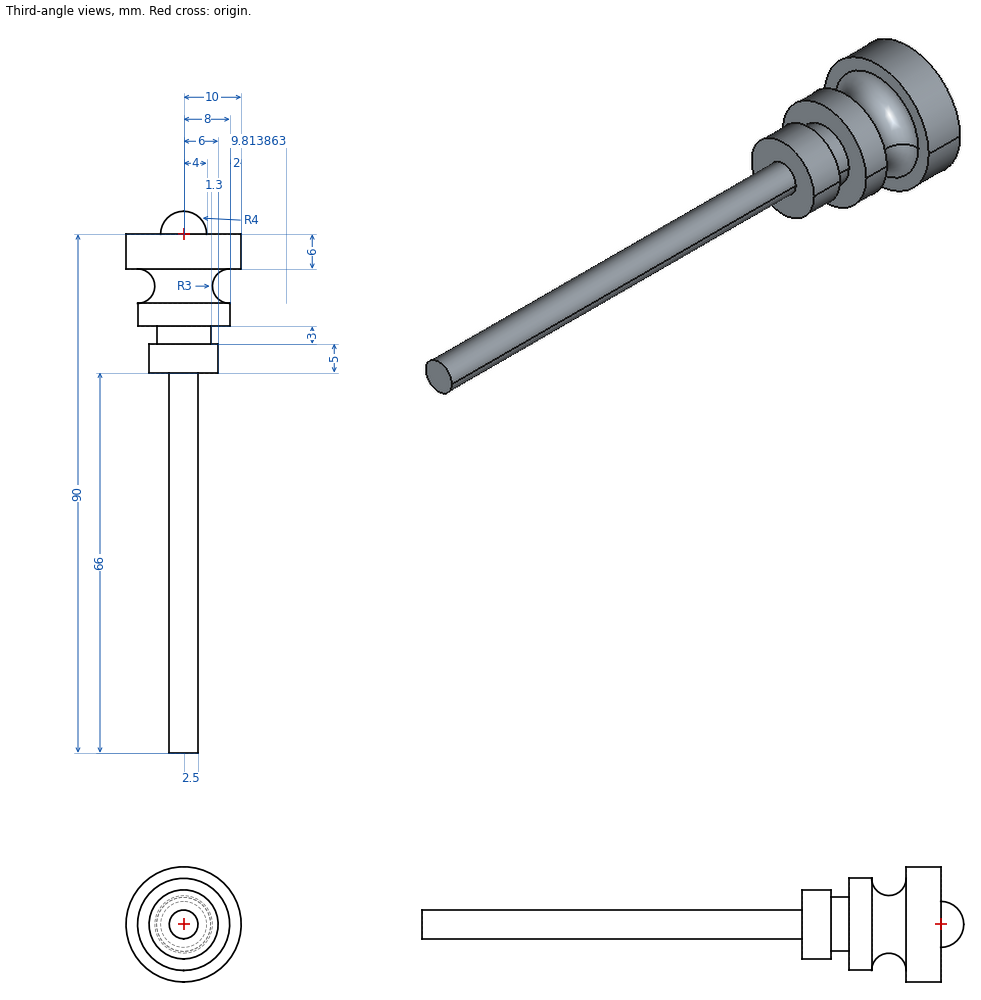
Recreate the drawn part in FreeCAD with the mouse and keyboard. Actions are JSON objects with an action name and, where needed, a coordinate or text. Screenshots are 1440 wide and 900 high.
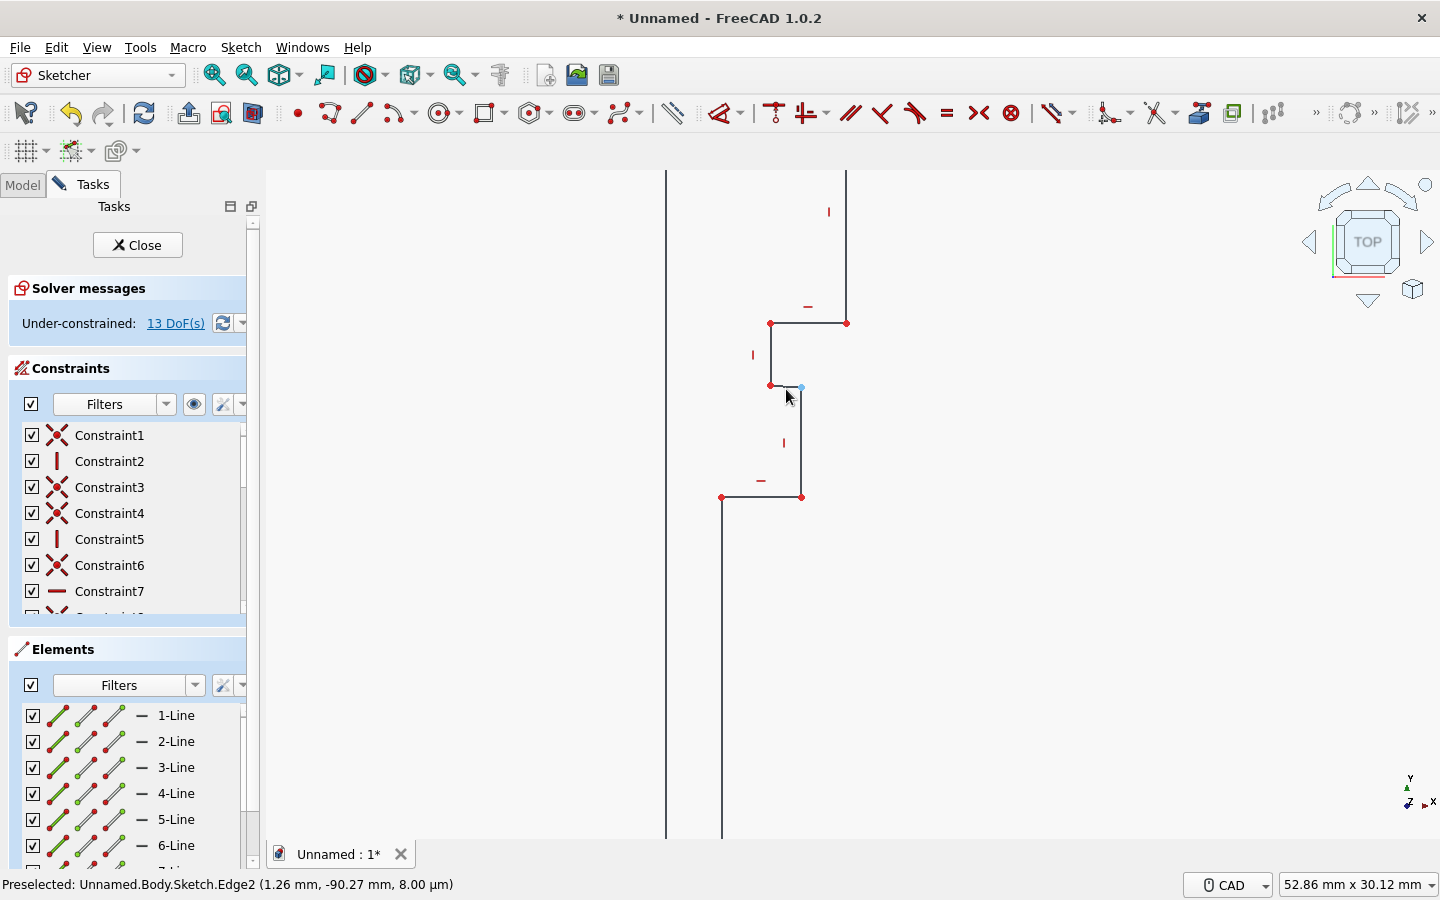
{"action": "left_click", "coordinate": [786, 387]}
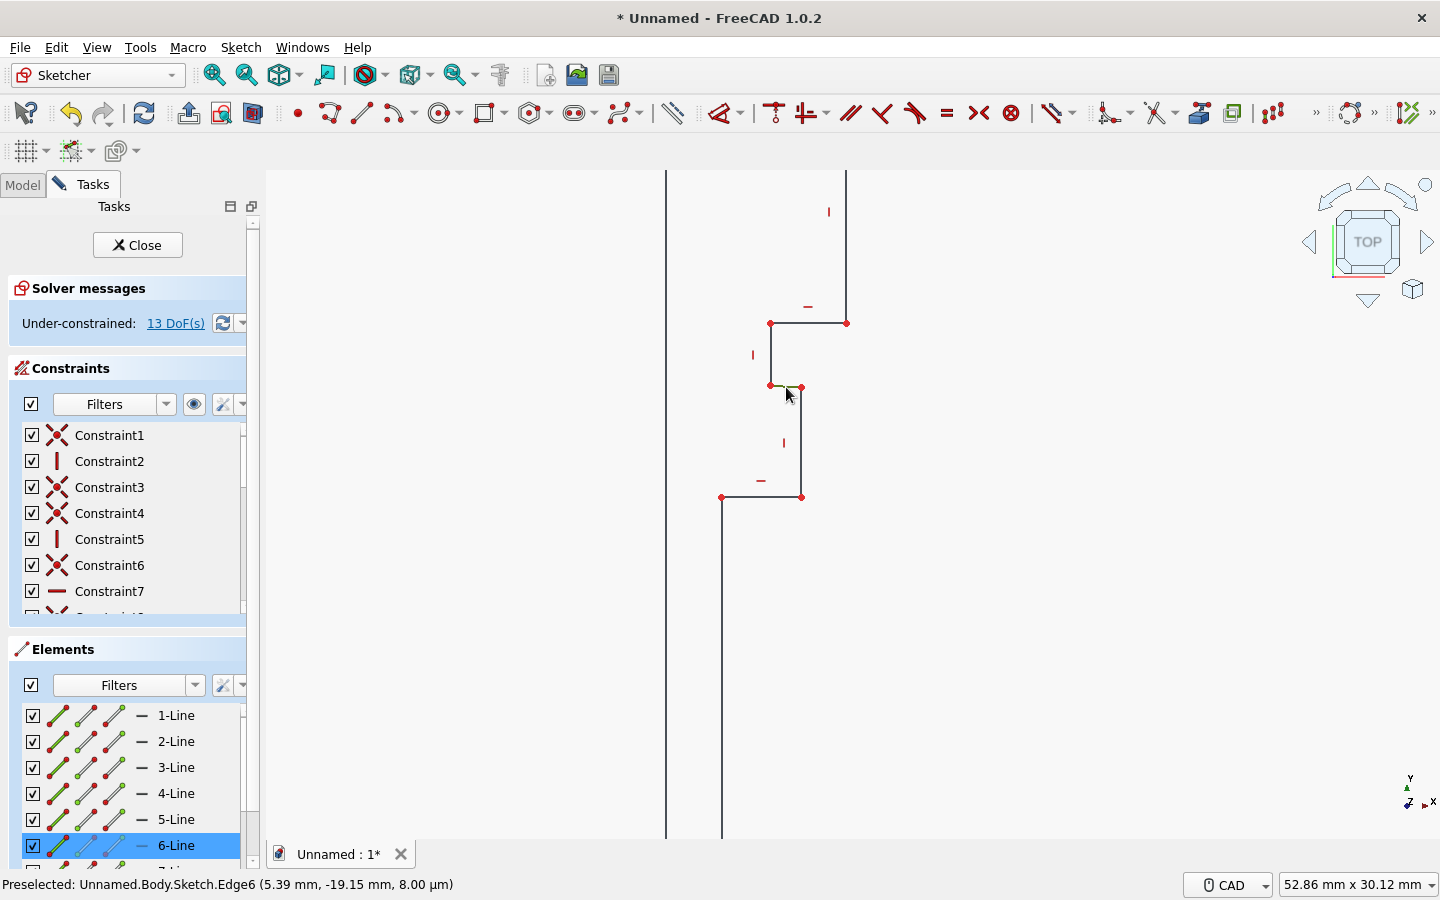
{"action": "left_click", "coordinate": [828, 114]}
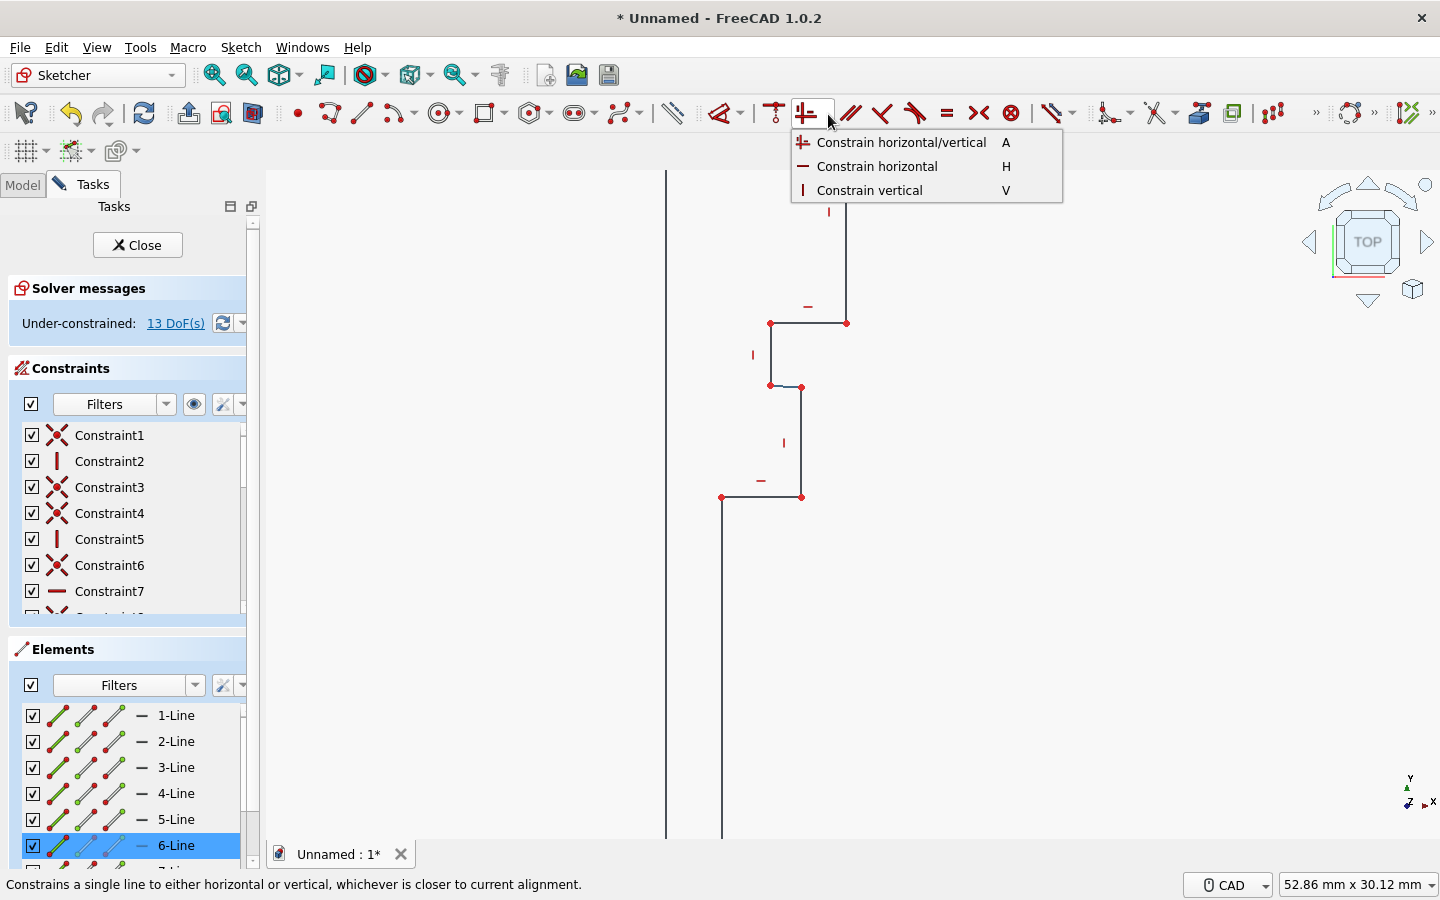
{"action": "left_click", "coordinate": [927, 166]}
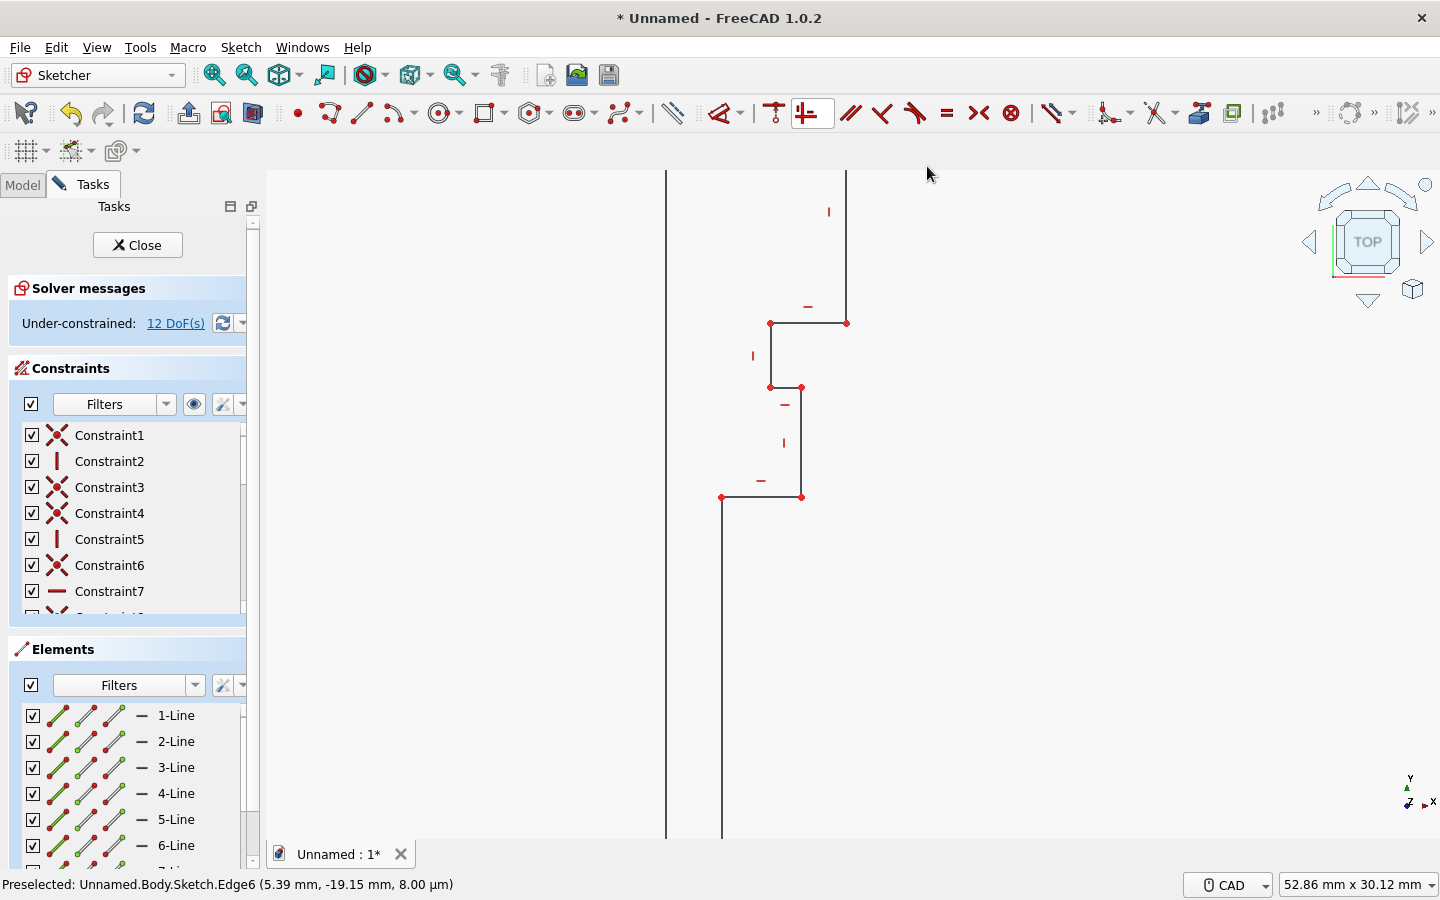
{"action": "scroll", "coordinate": [786, 389], "scroll_direction": "down", "scroll_amount": 8}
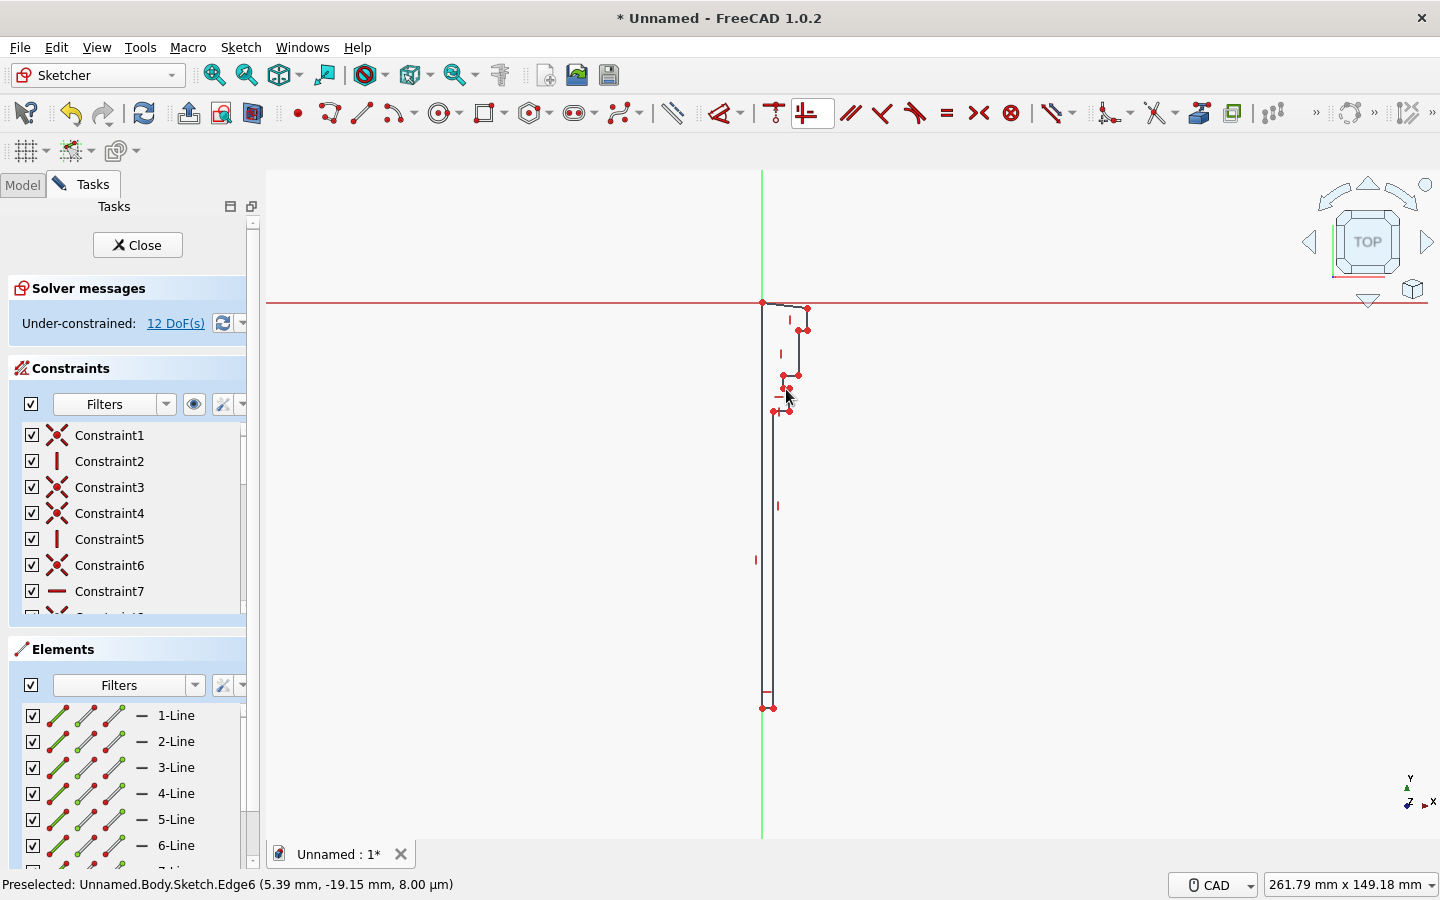
{"action": "scroll", "coordinate": [801, 331], "scroll_direction": "up", "scroll_amount": 9}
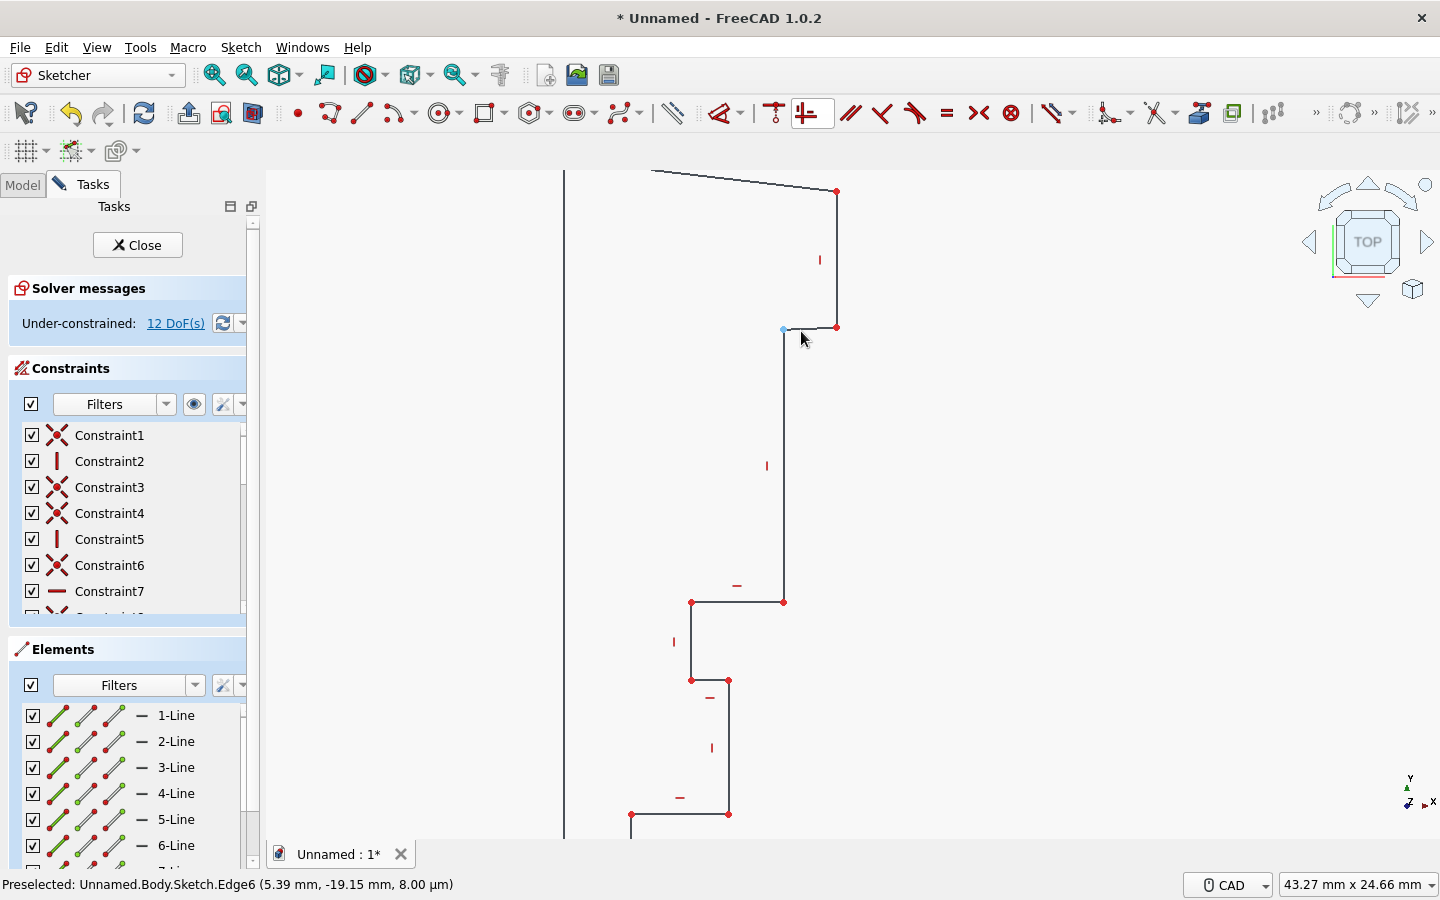
{"action": "left_click", "coordinate": [800, 329]}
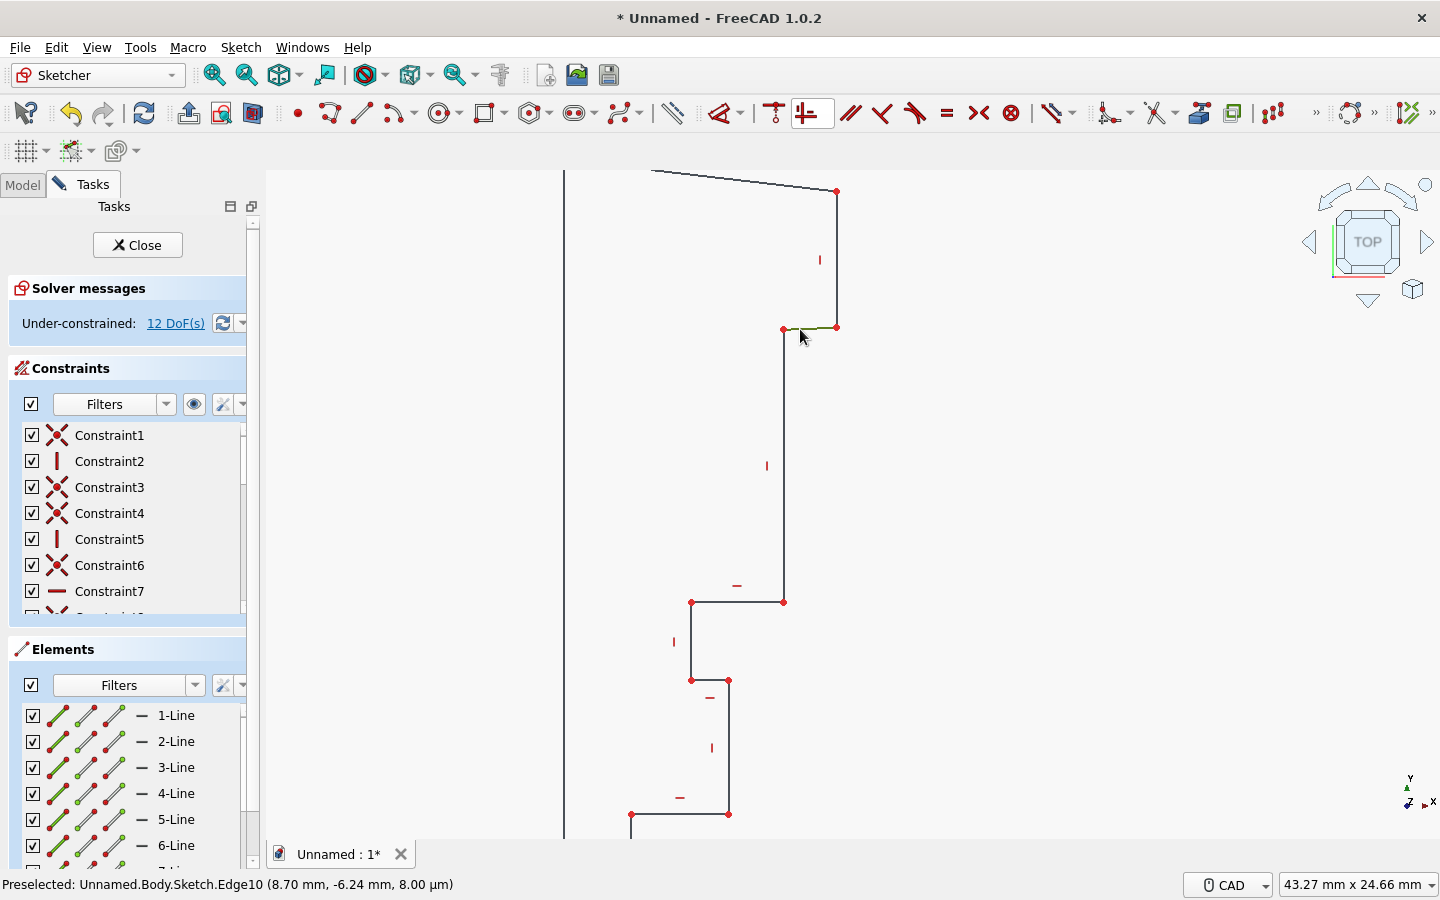
{"action": "key", "text": "h"}